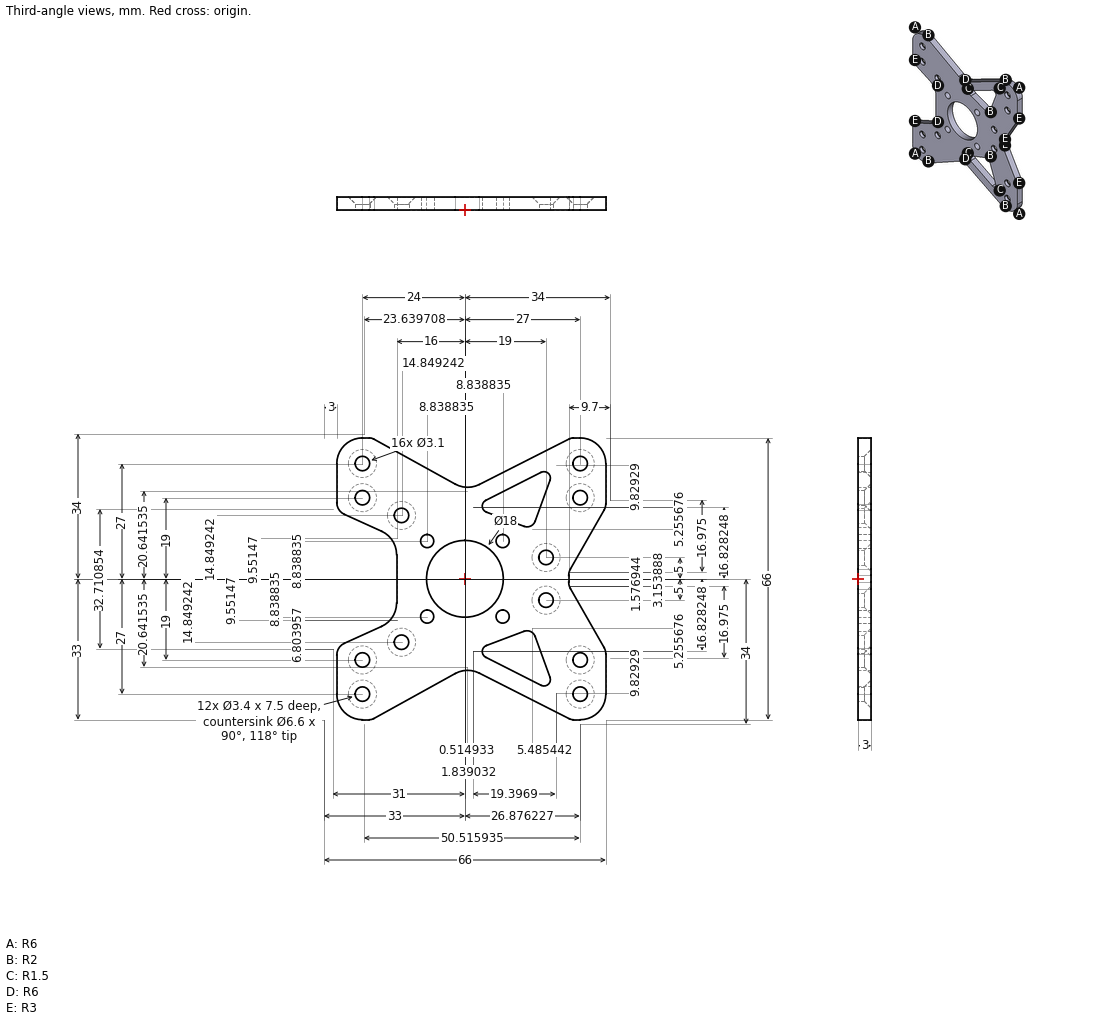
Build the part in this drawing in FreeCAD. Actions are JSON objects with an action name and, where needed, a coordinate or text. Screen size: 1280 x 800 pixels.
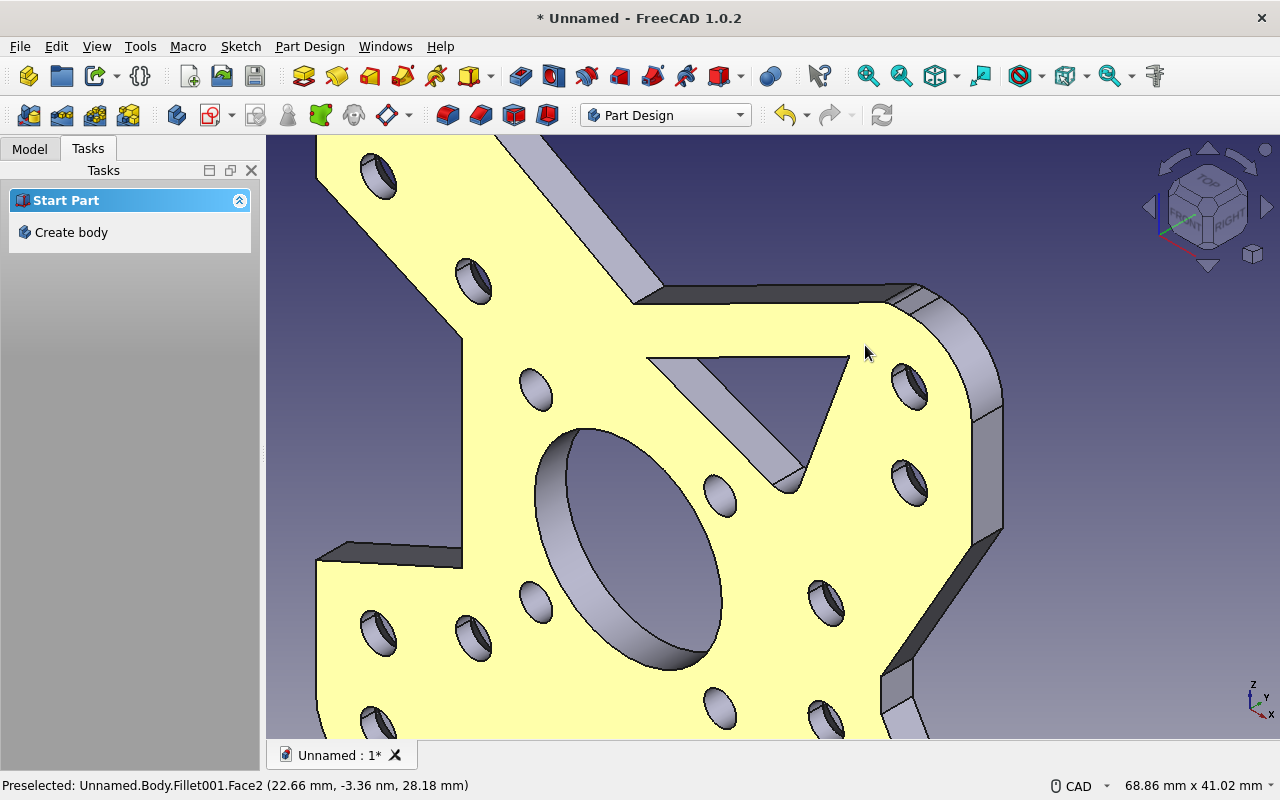
{"action": "left_click", "coordinate": [869, 76]}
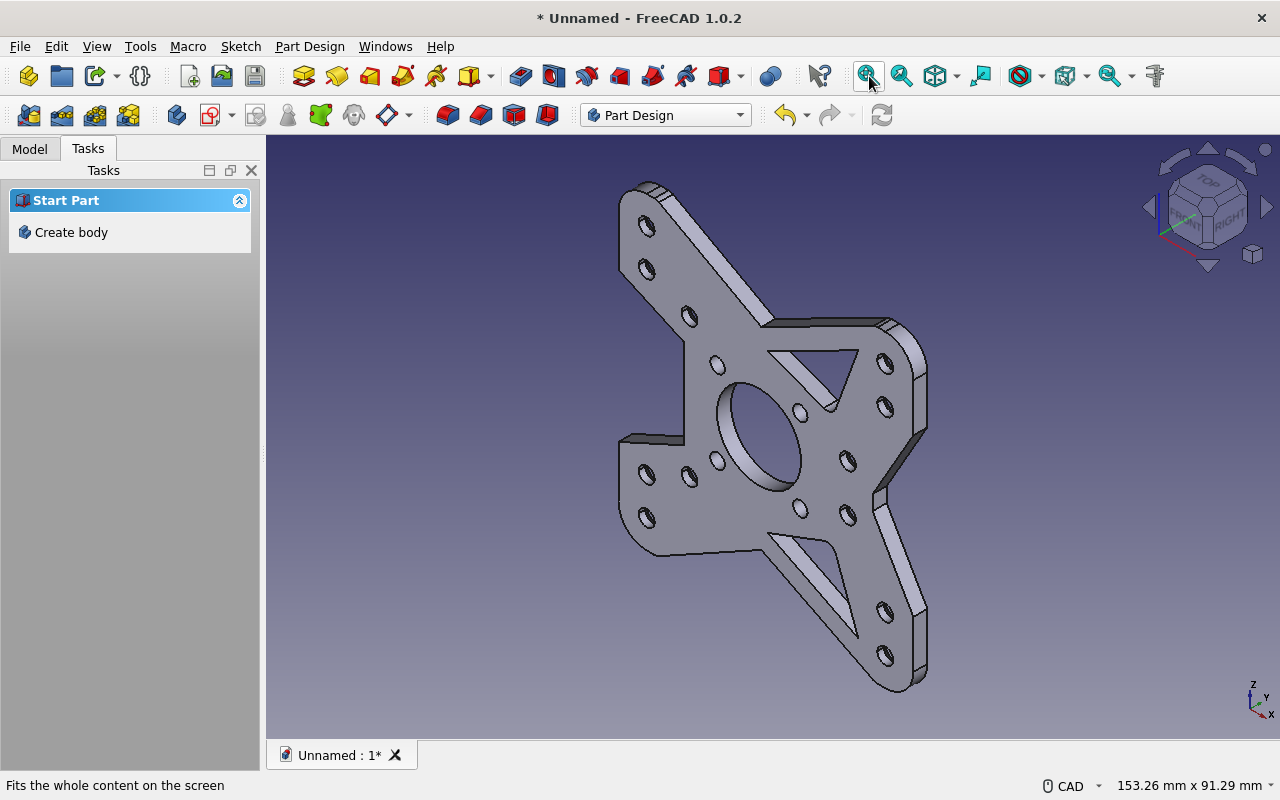
{"action": "key", "text": "1"}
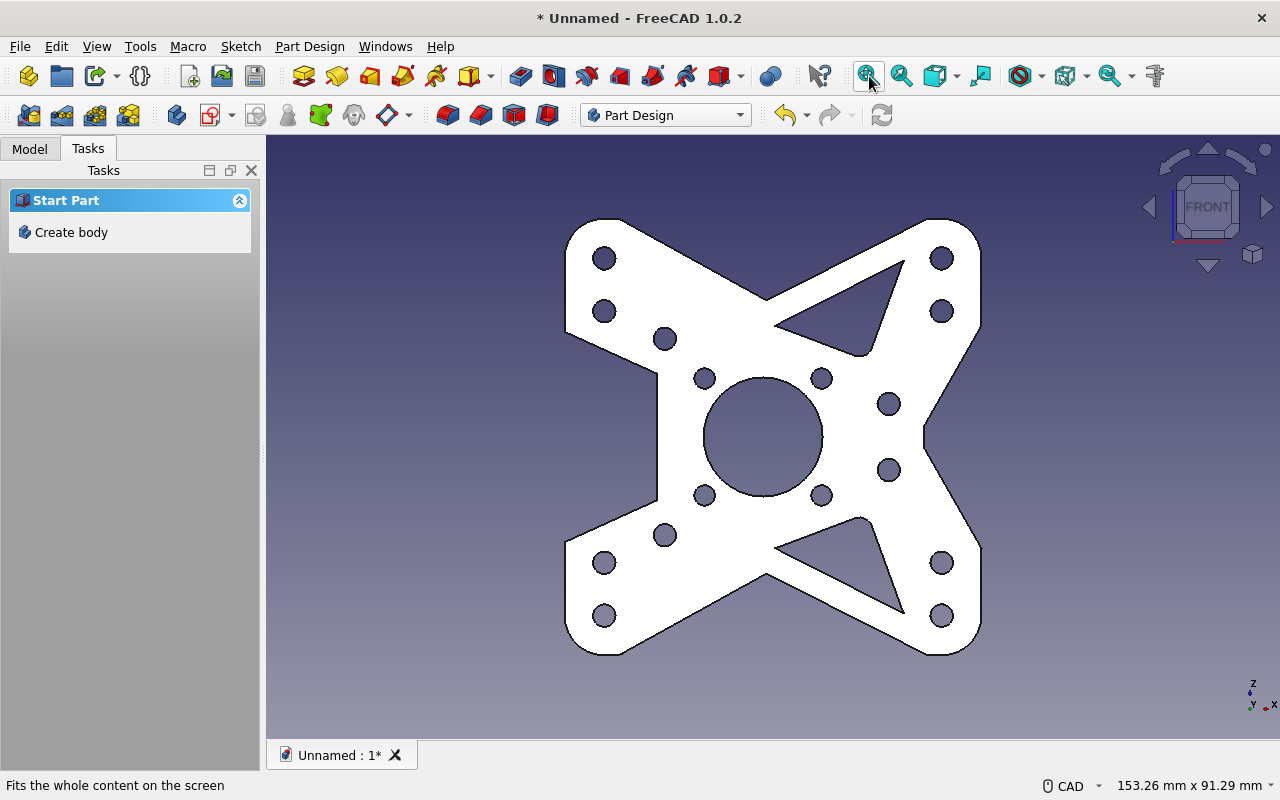
{"action": "scroll", "coordinate": [904, 260], "scroll_direction": "up", "scroll_amount": 4}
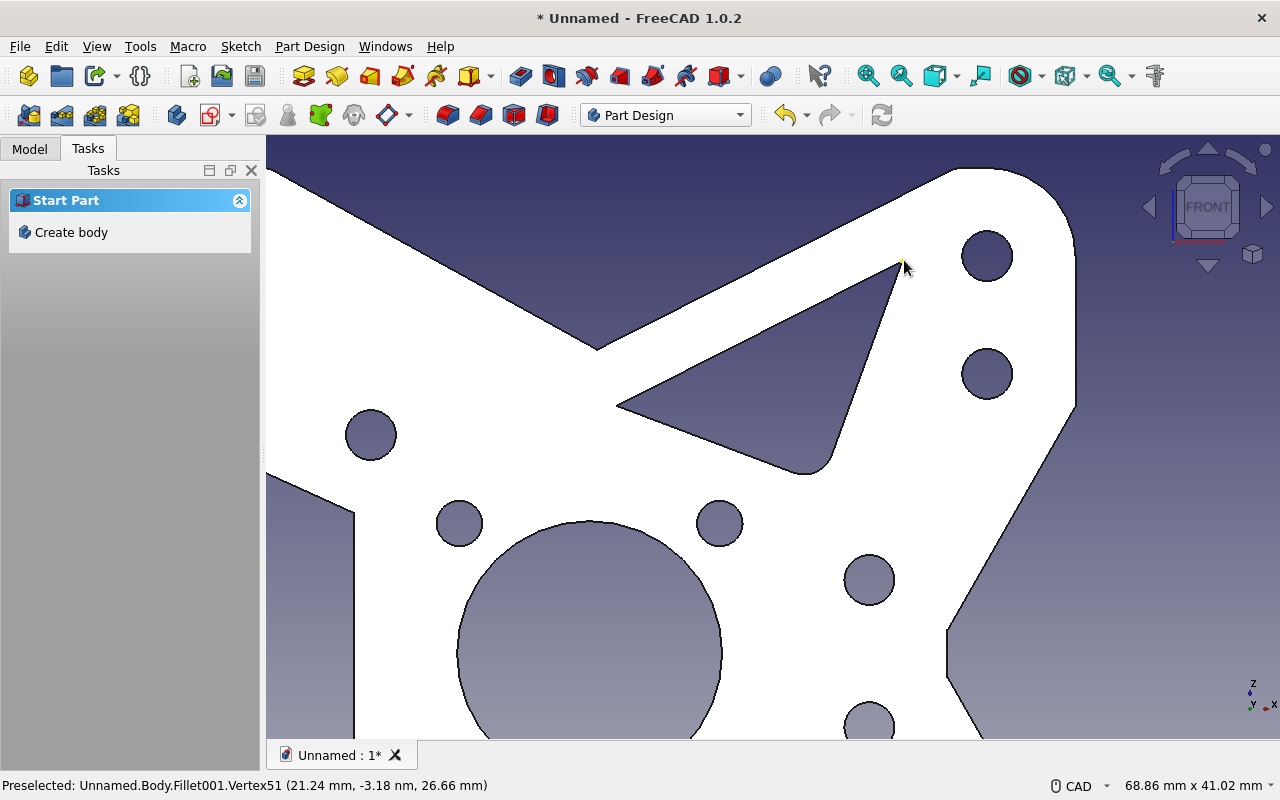
{"action": "left_click", "coordinate": [869, 76]}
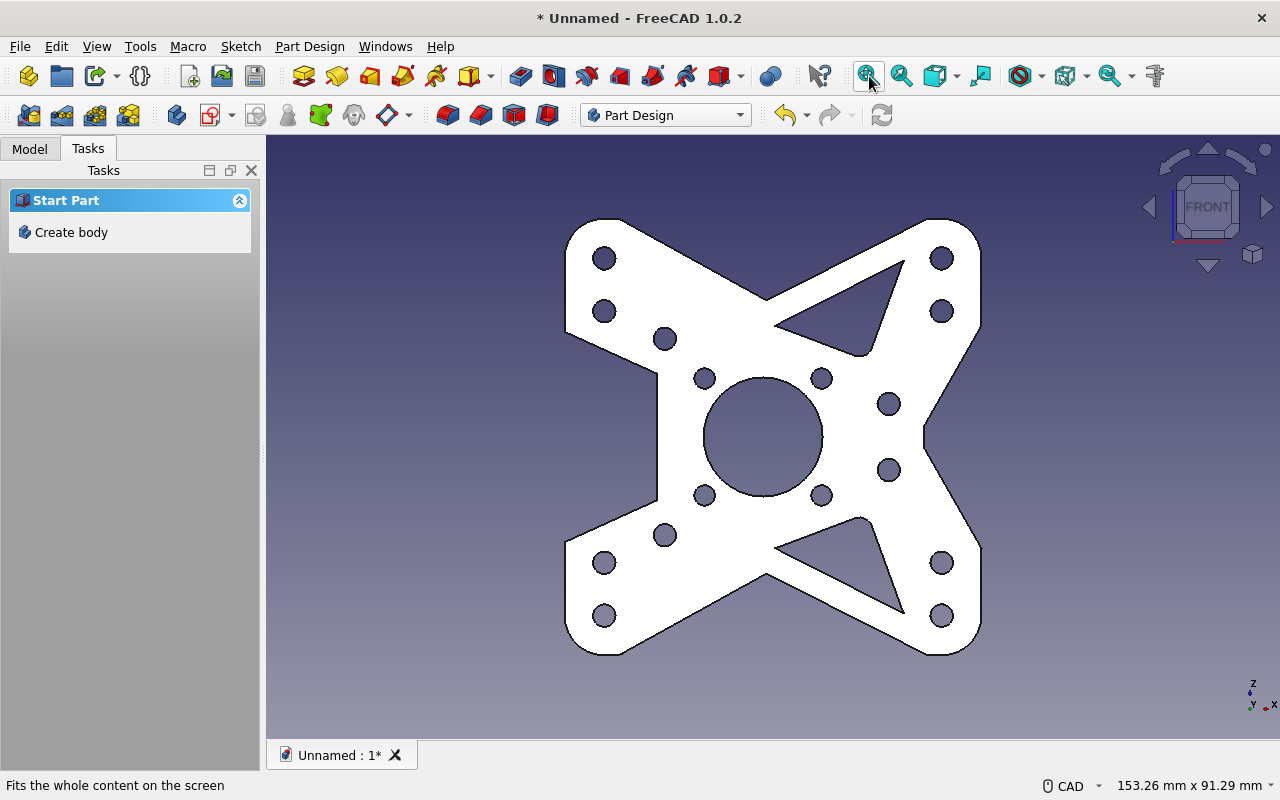
{"action": "key", "text": "3"}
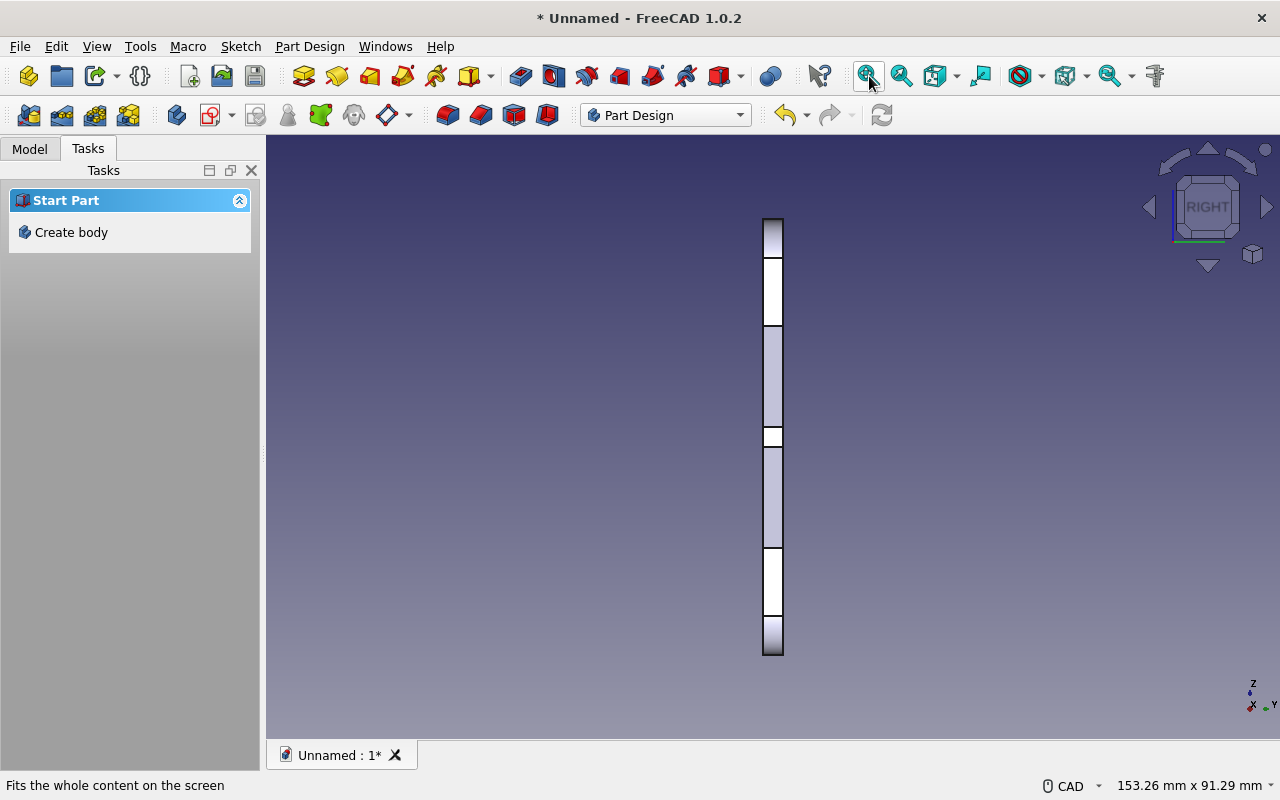
{"action": "scroll", "coordinate": [773, 260], "scroll_direction": "up", "scroll_amount": 4}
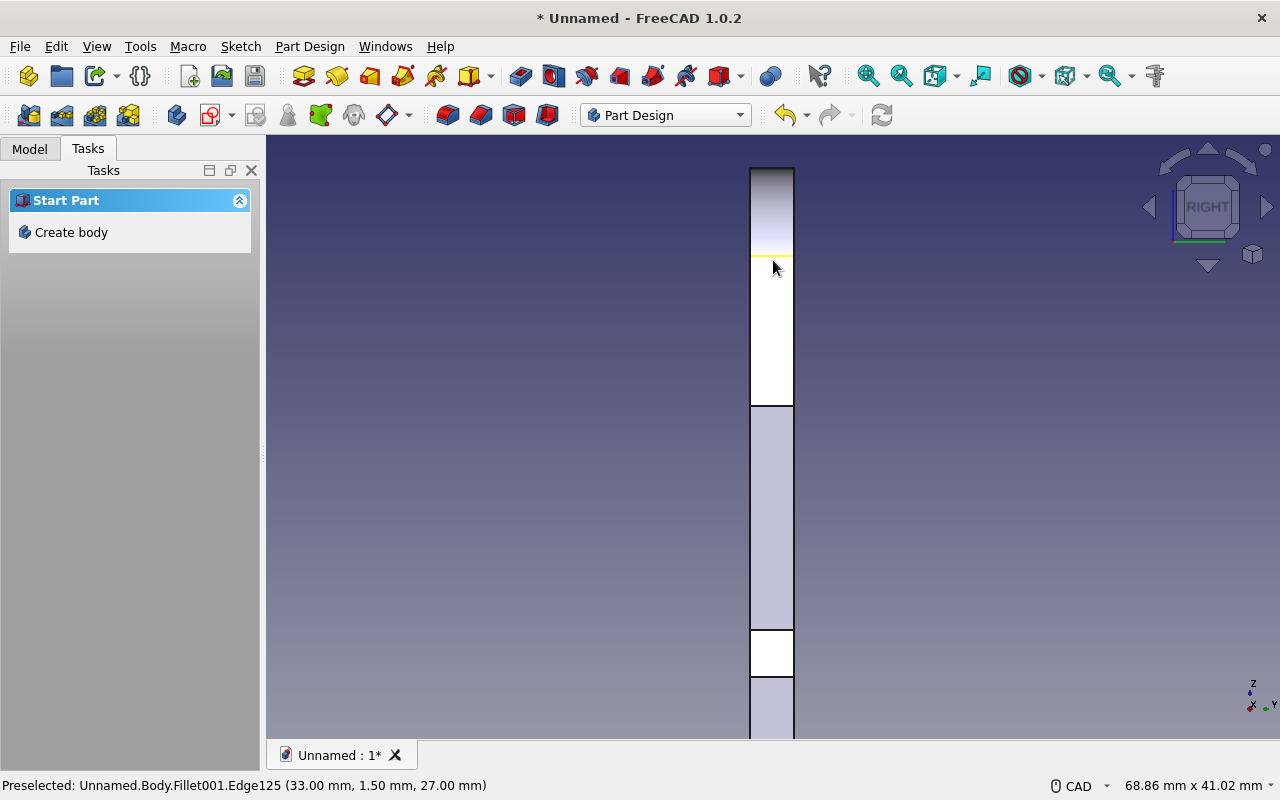
{"action": "left_click", "coordinate": [869, 76]}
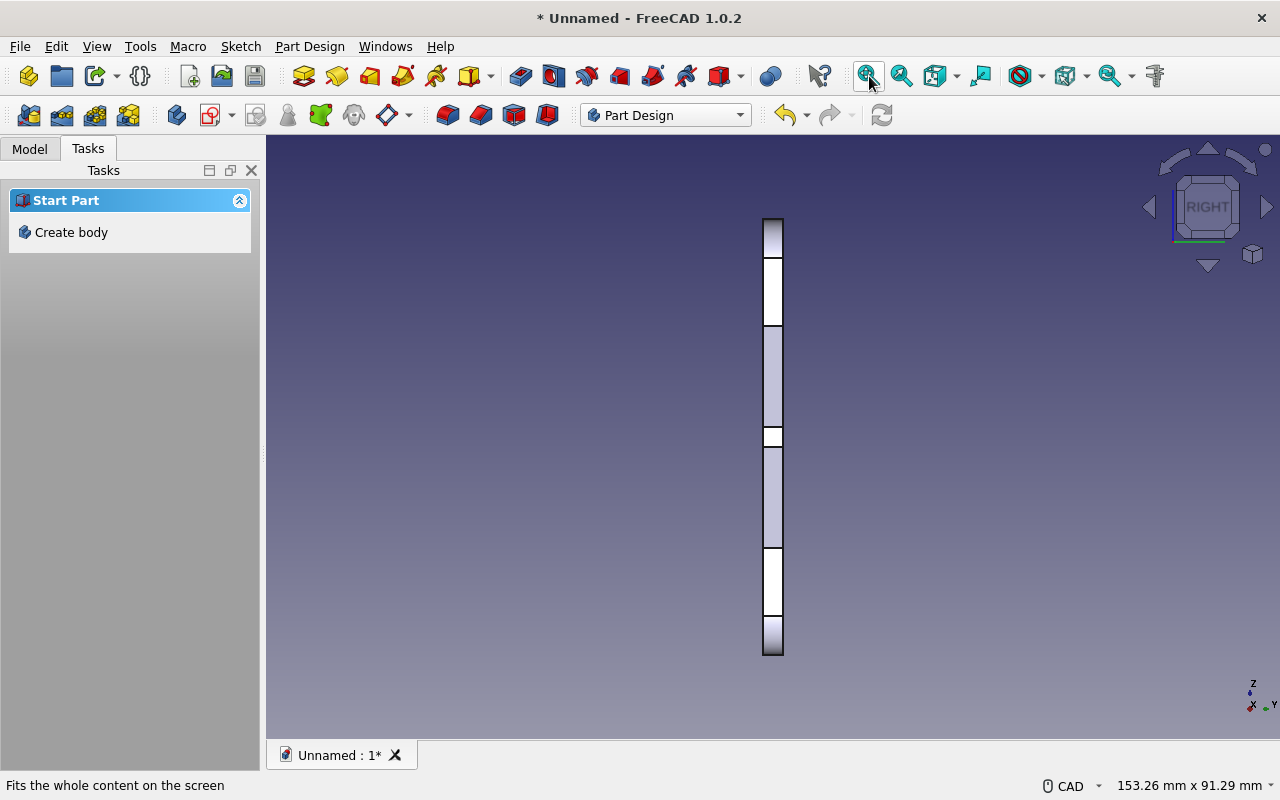
{"action": "key", "text": "5"}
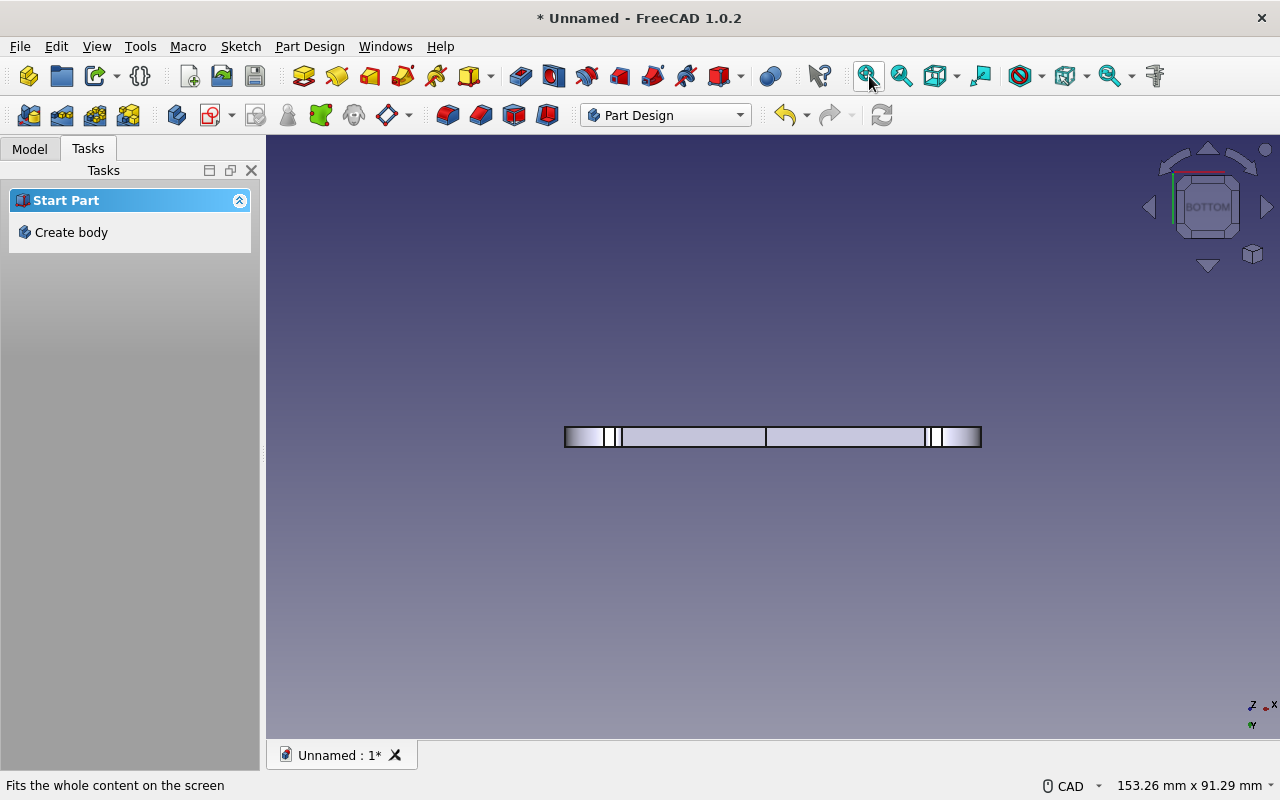
{"action": "key", "text": "v f"}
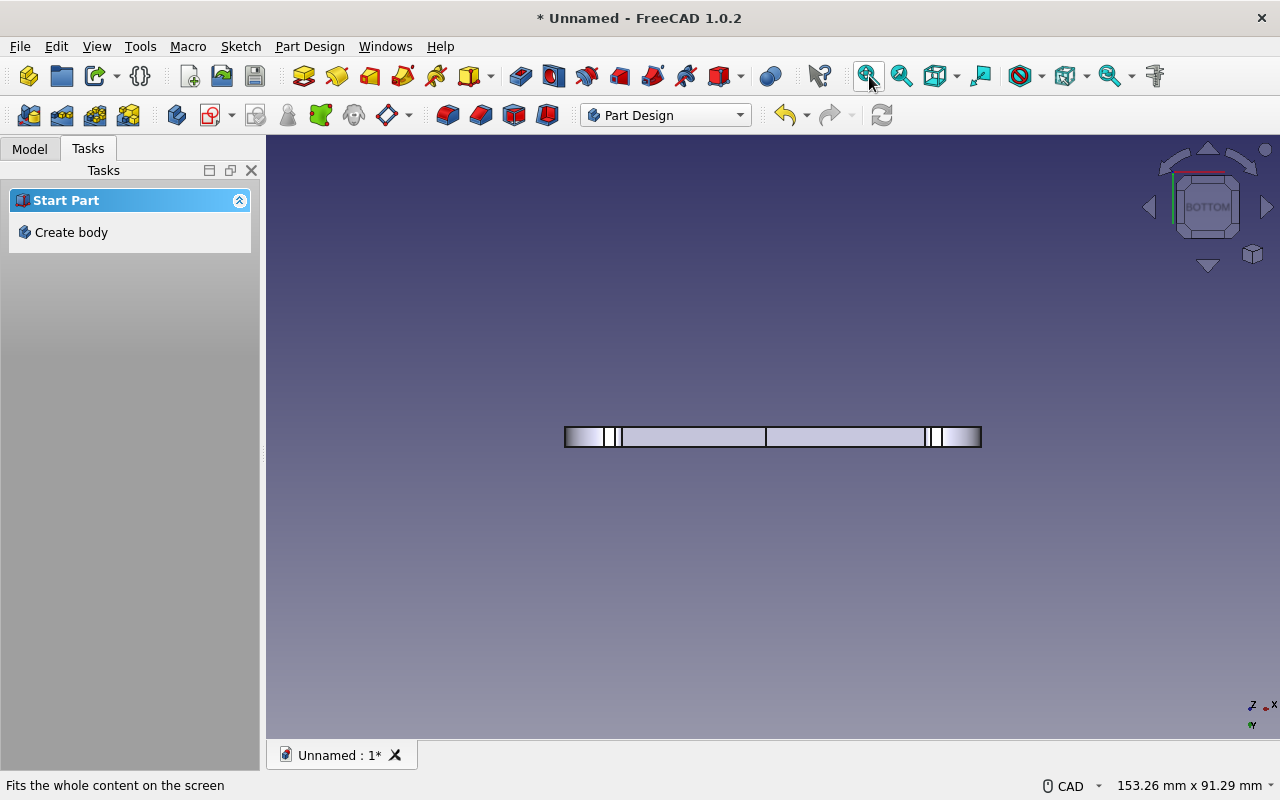
{"action": "scroll", "coordinate": [904, 436], "scroll_direction": "up", "scroll_amount": 4}